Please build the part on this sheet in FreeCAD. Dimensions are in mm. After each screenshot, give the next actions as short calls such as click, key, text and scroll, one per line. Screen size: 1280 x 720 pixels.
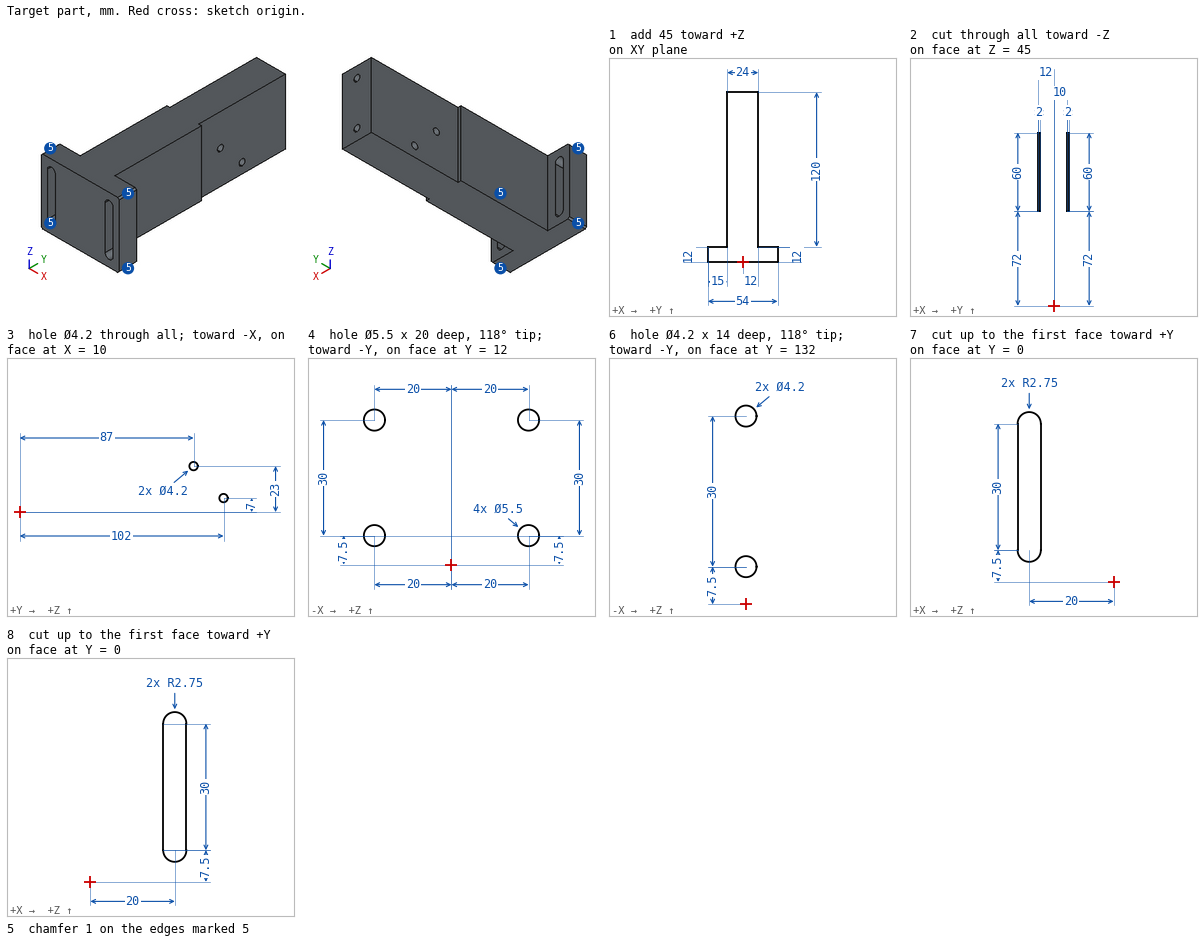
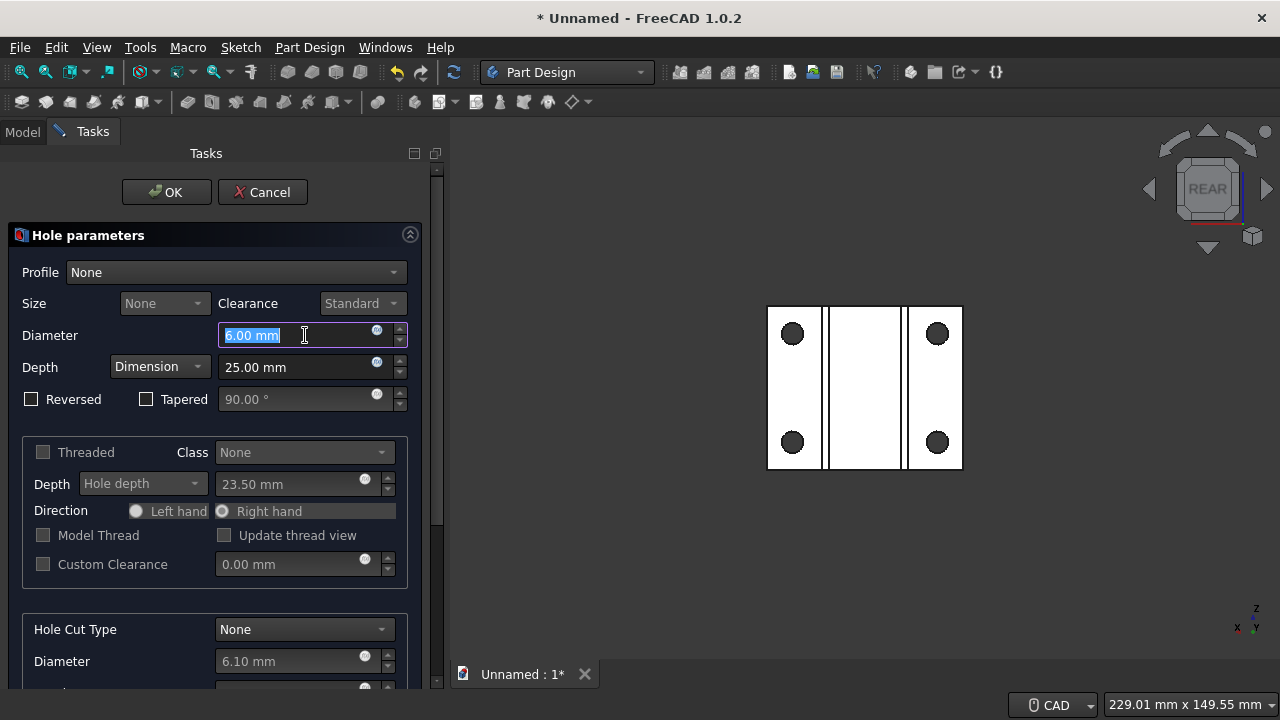
text(5.5)
key(Tab)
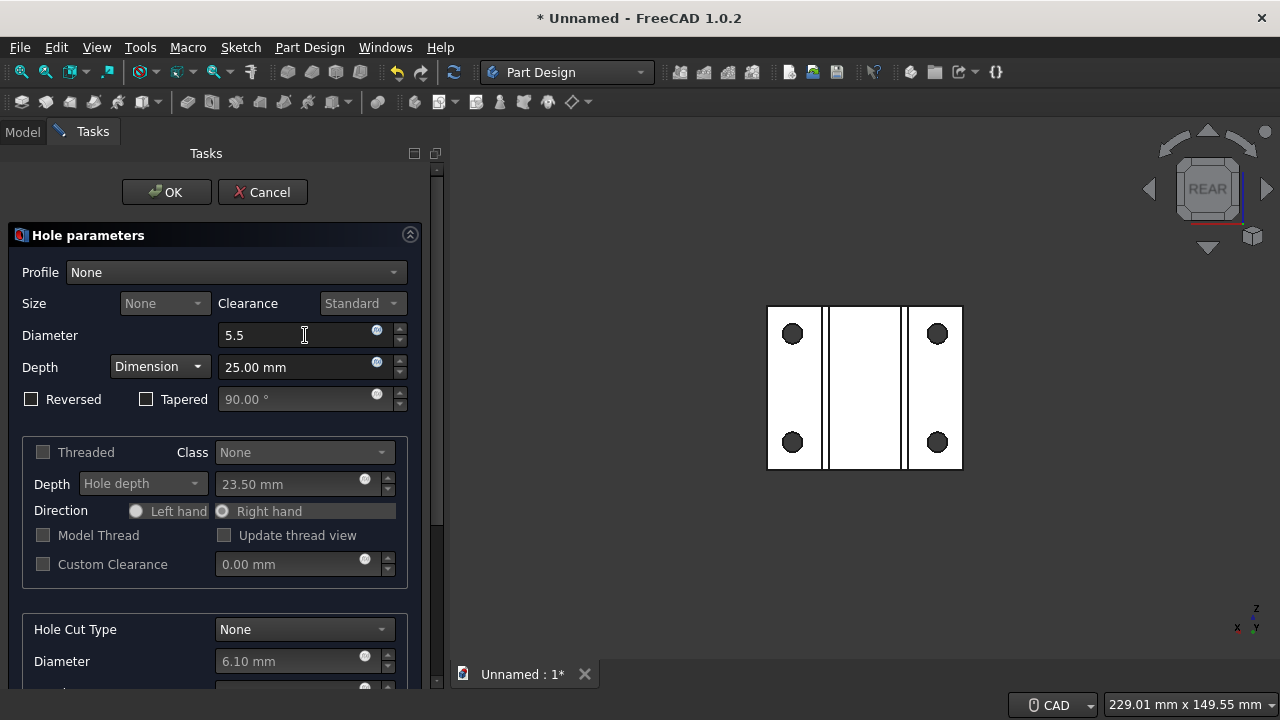
triple_click(305, 367)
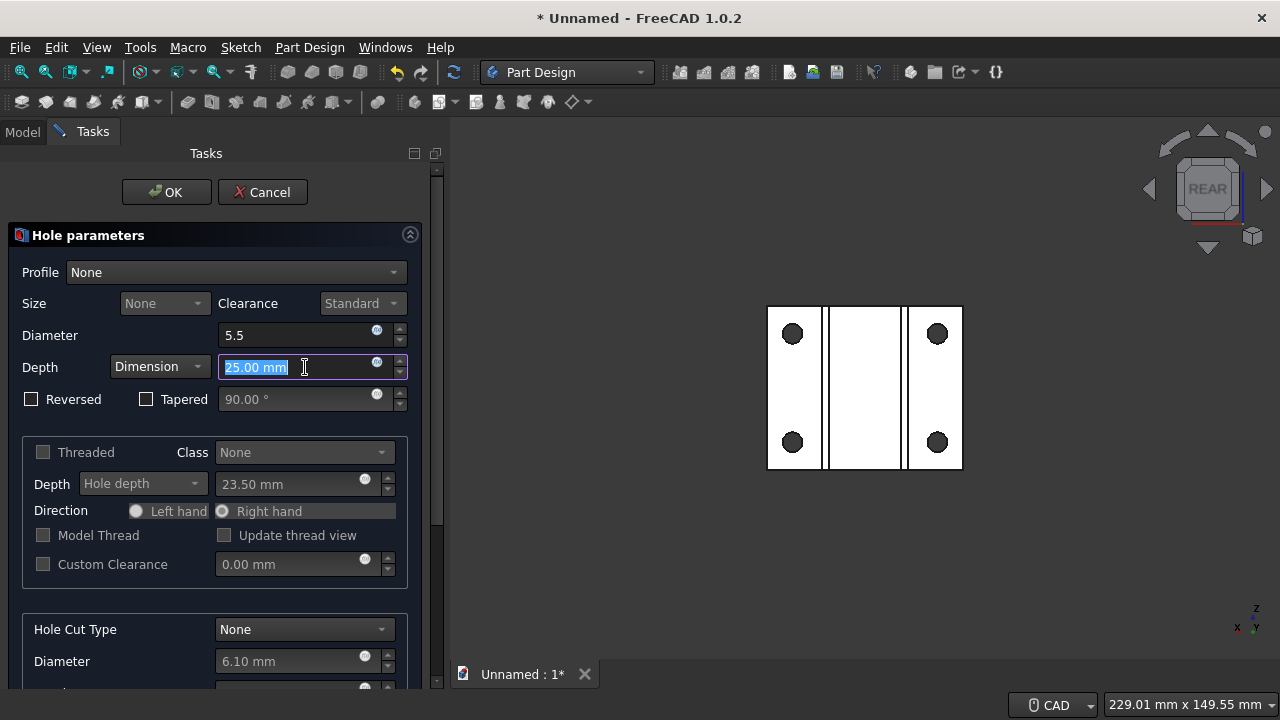
text(20)
key(Tab)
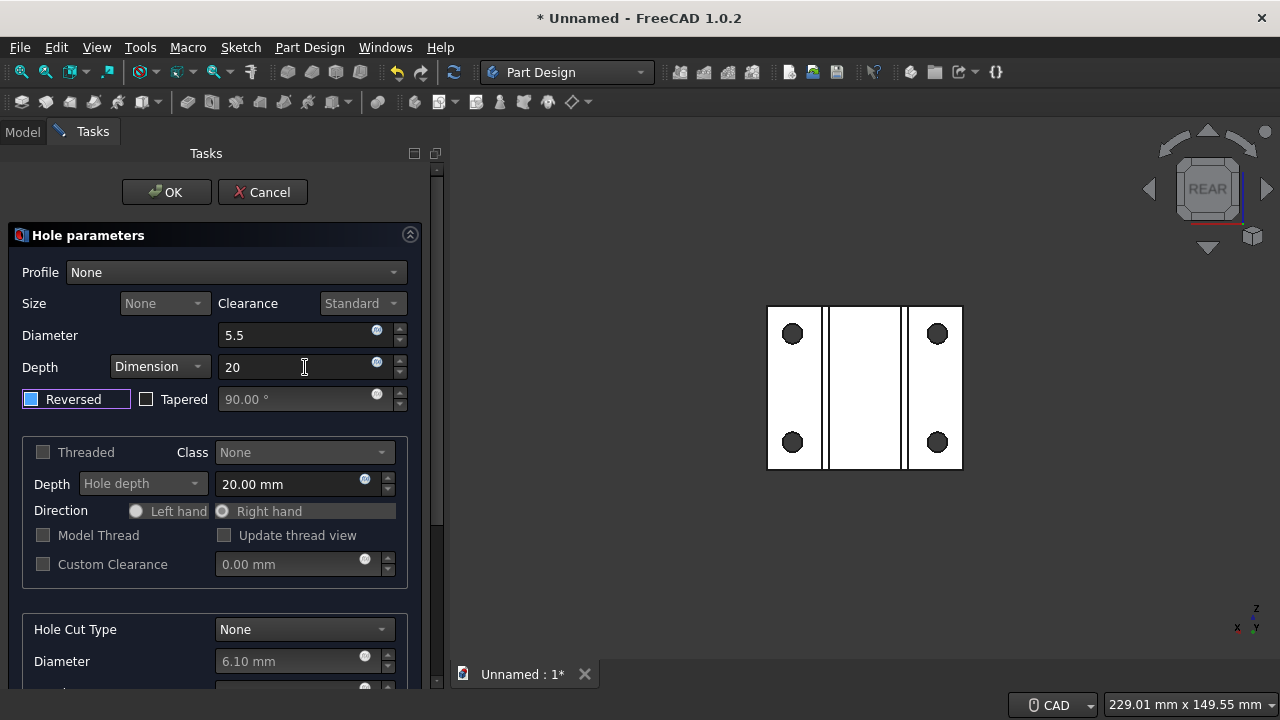
click(167, 192)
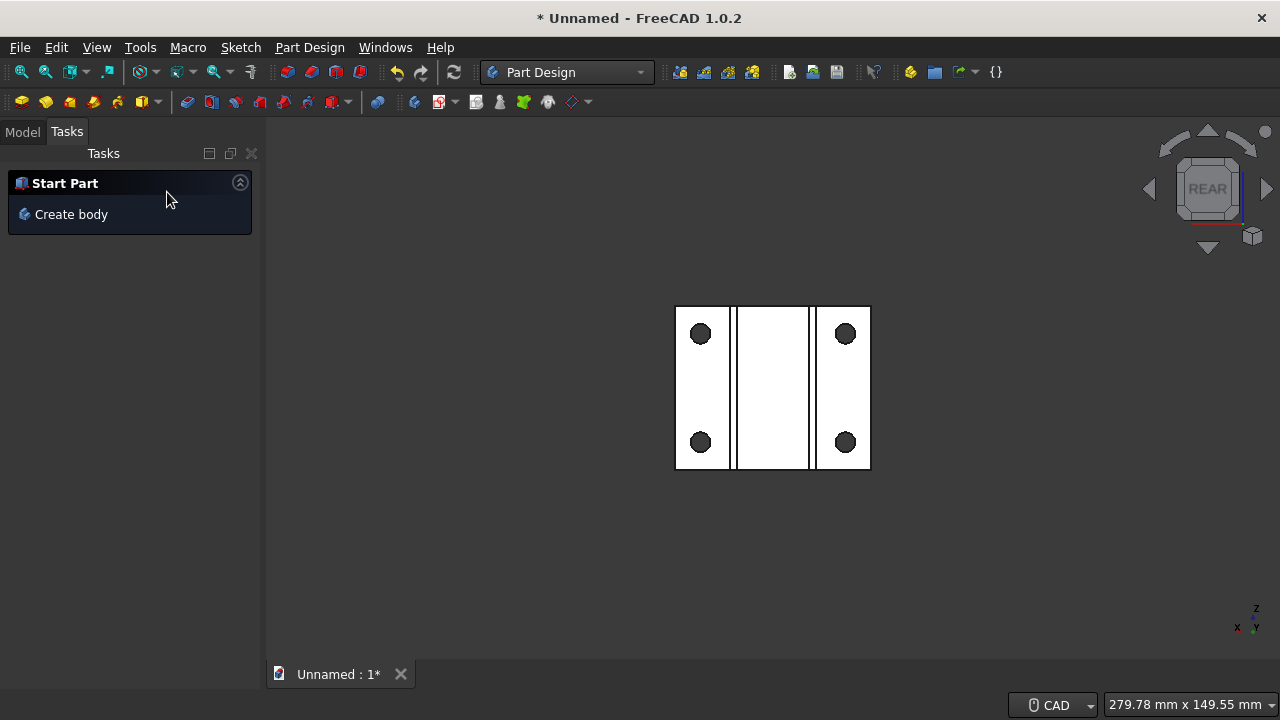
click(22, 72)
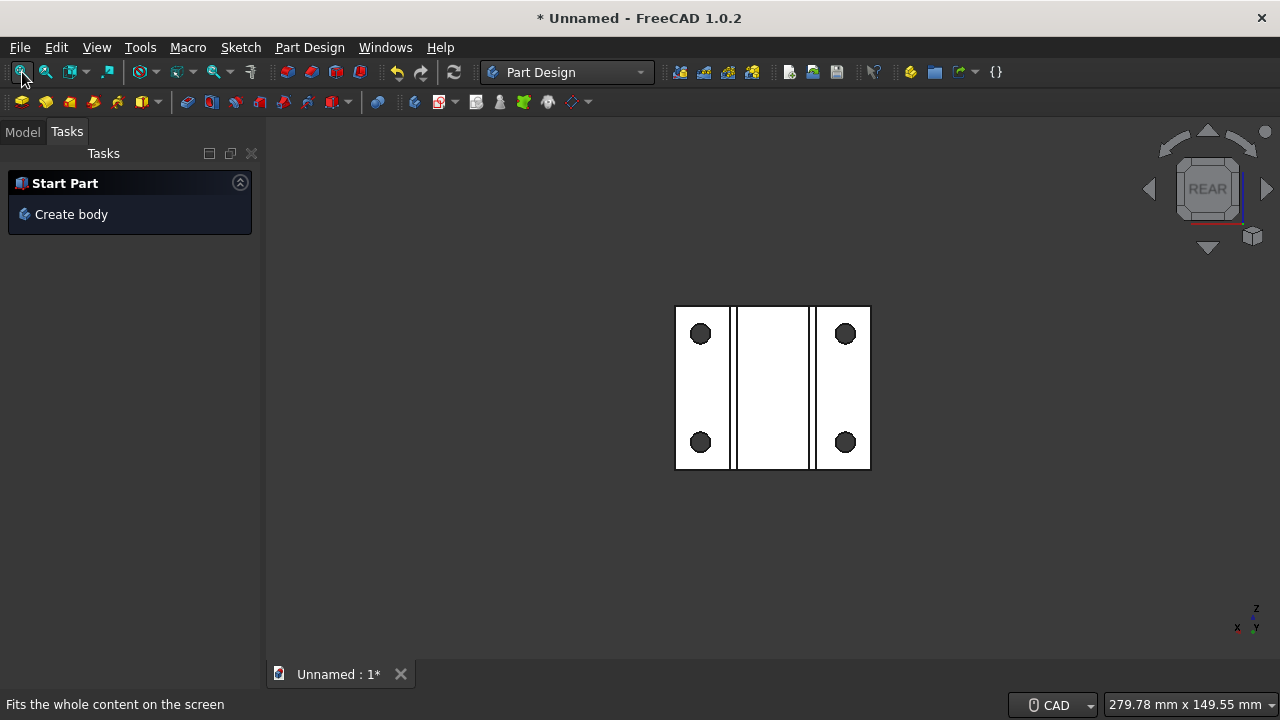
key(0)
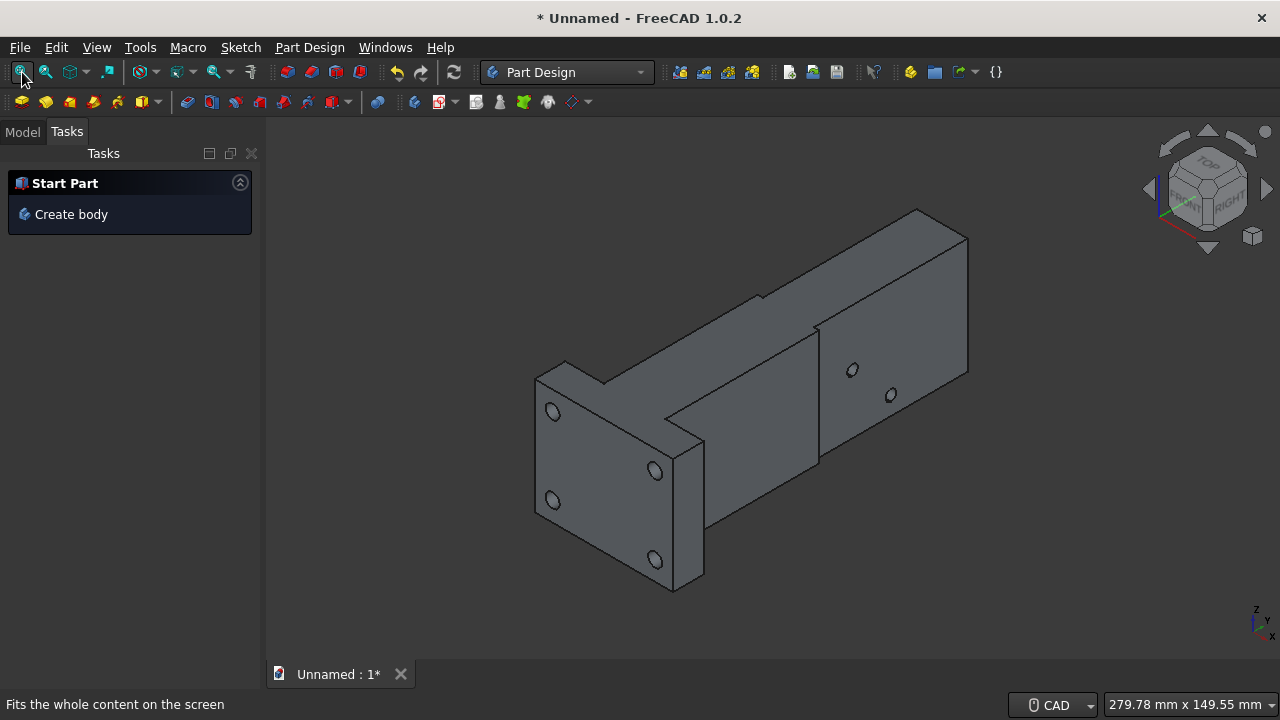
click(688, 449)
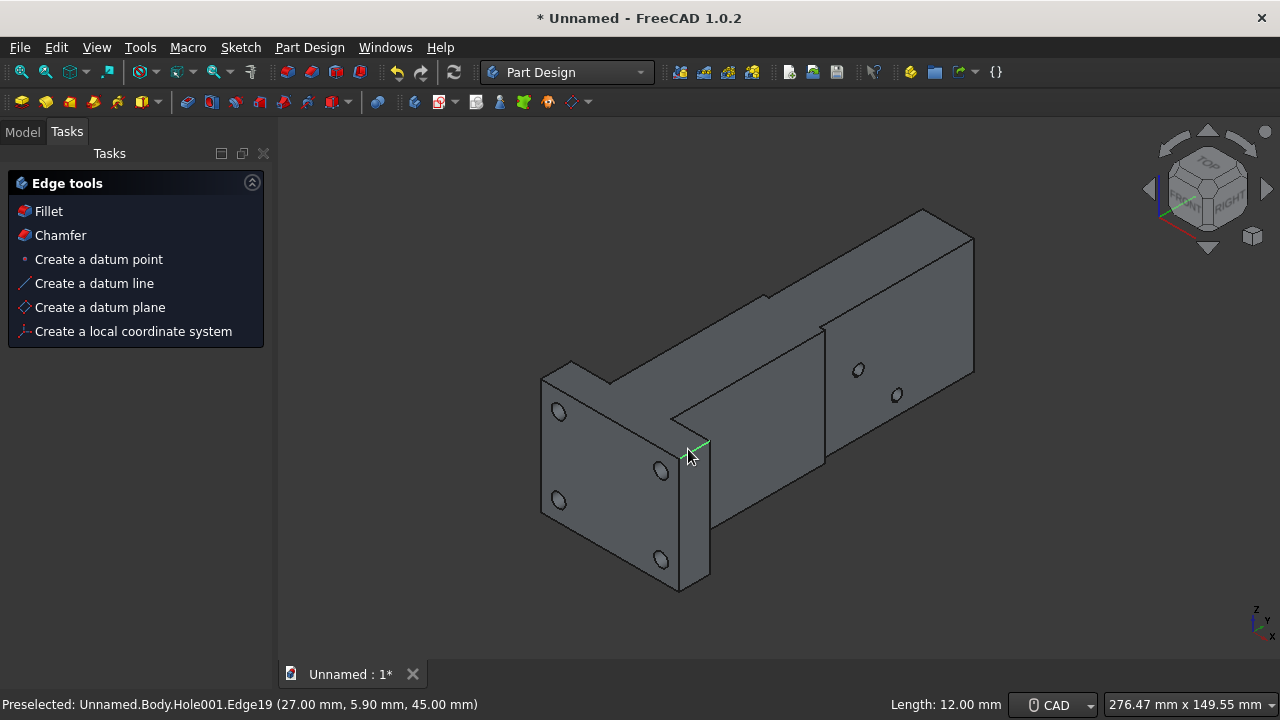
key(2)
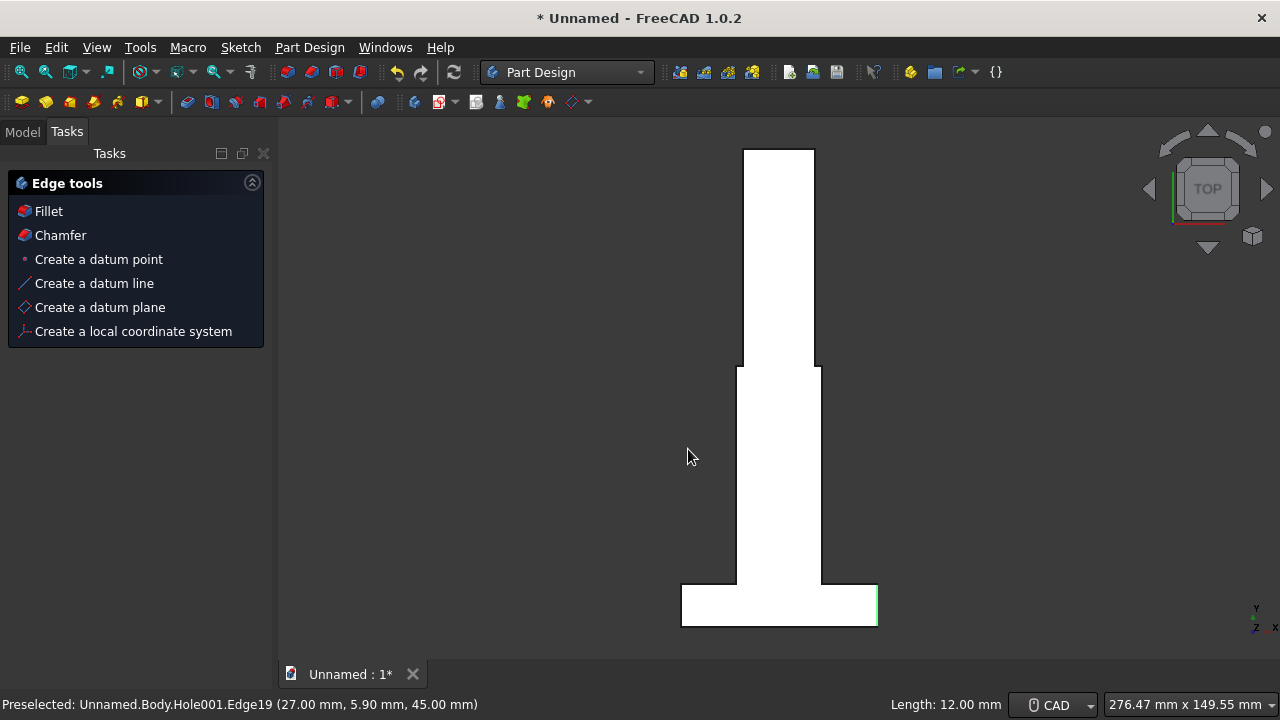
click(681, 604, ctrl)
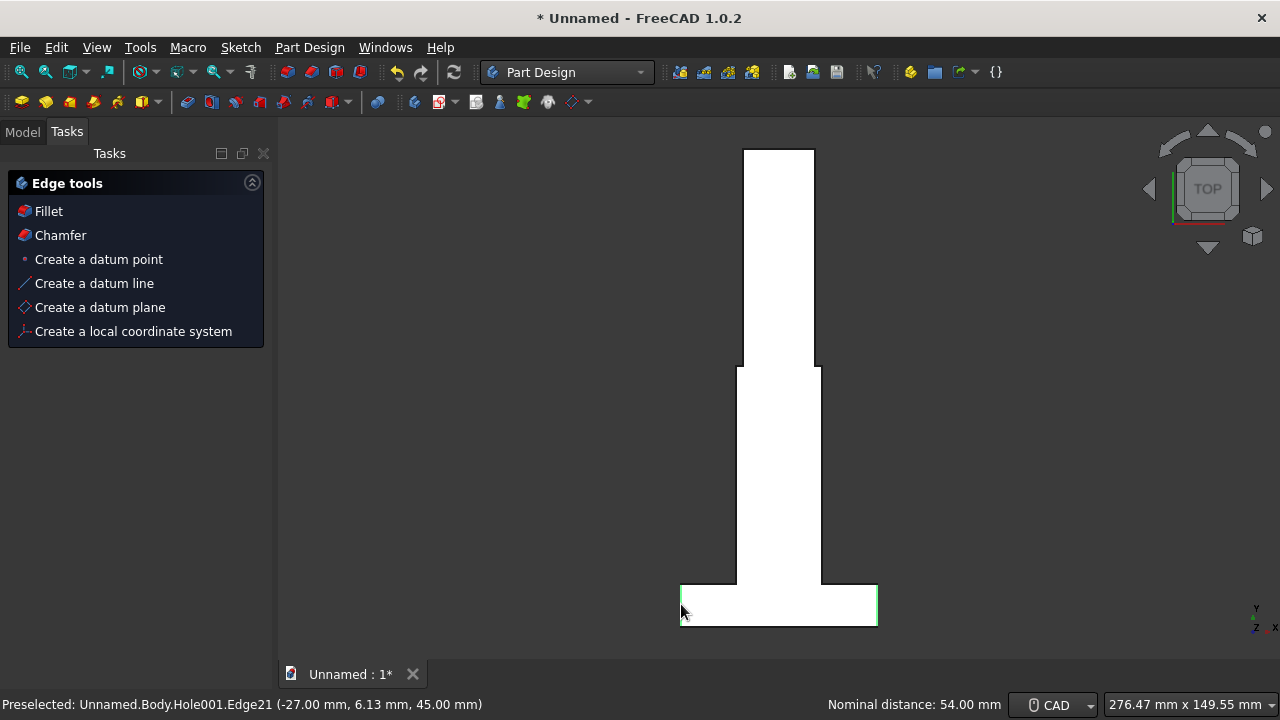
key(1)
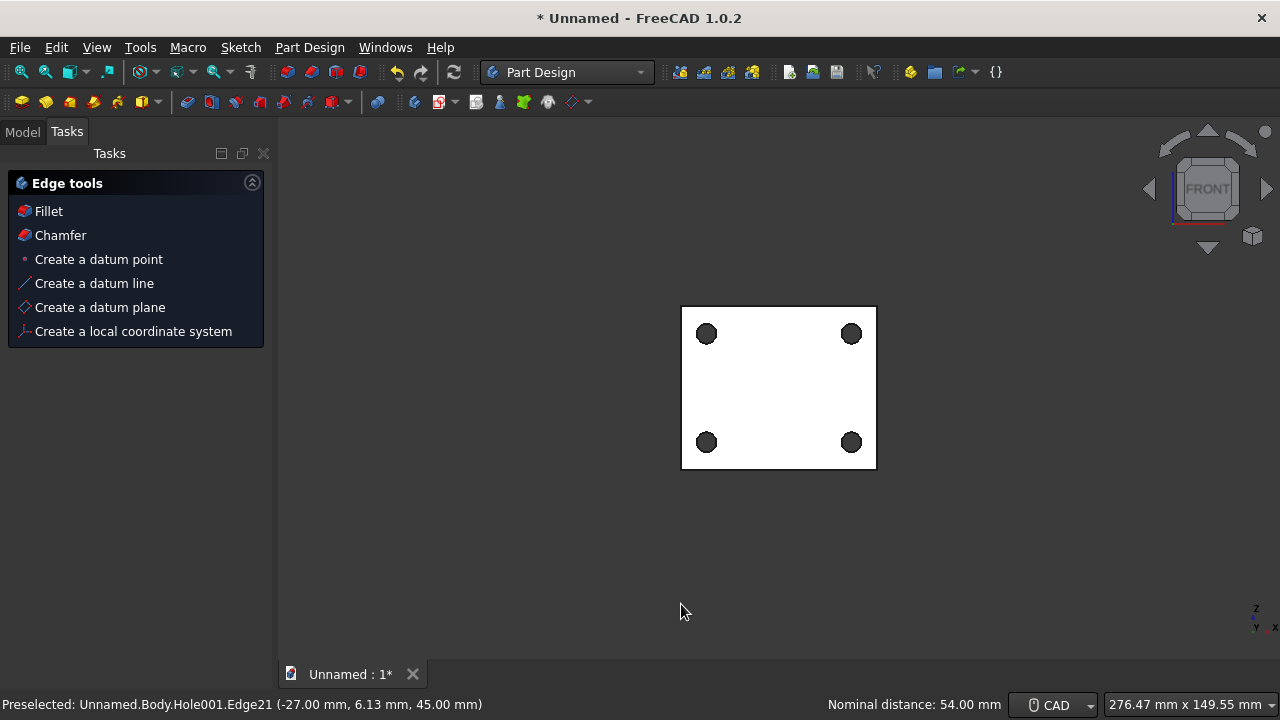
click(22, 72)